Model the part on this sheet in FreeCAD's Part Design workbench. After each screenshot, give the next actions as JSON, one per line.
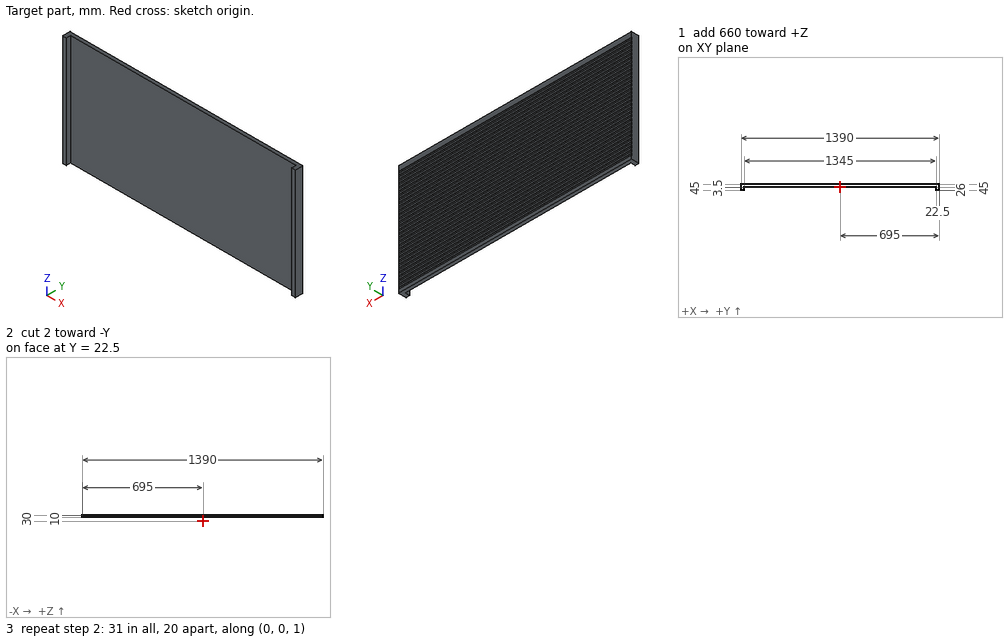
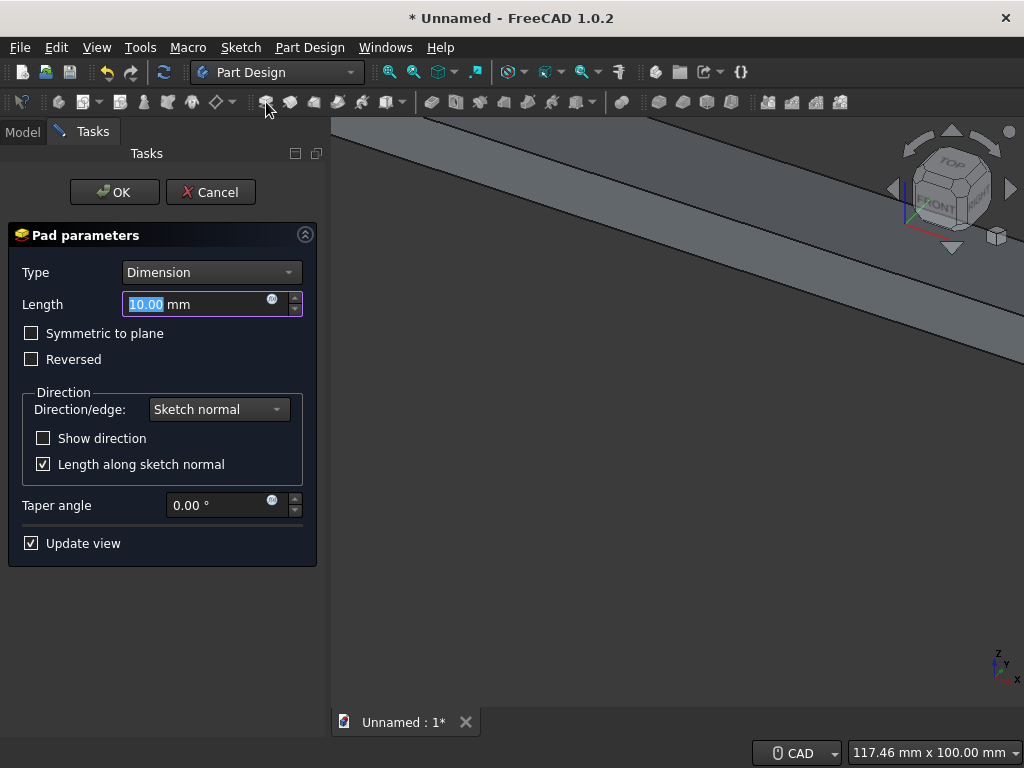
{"action": "type", "text": "660"}
{"action": "key", "text": "Tab"}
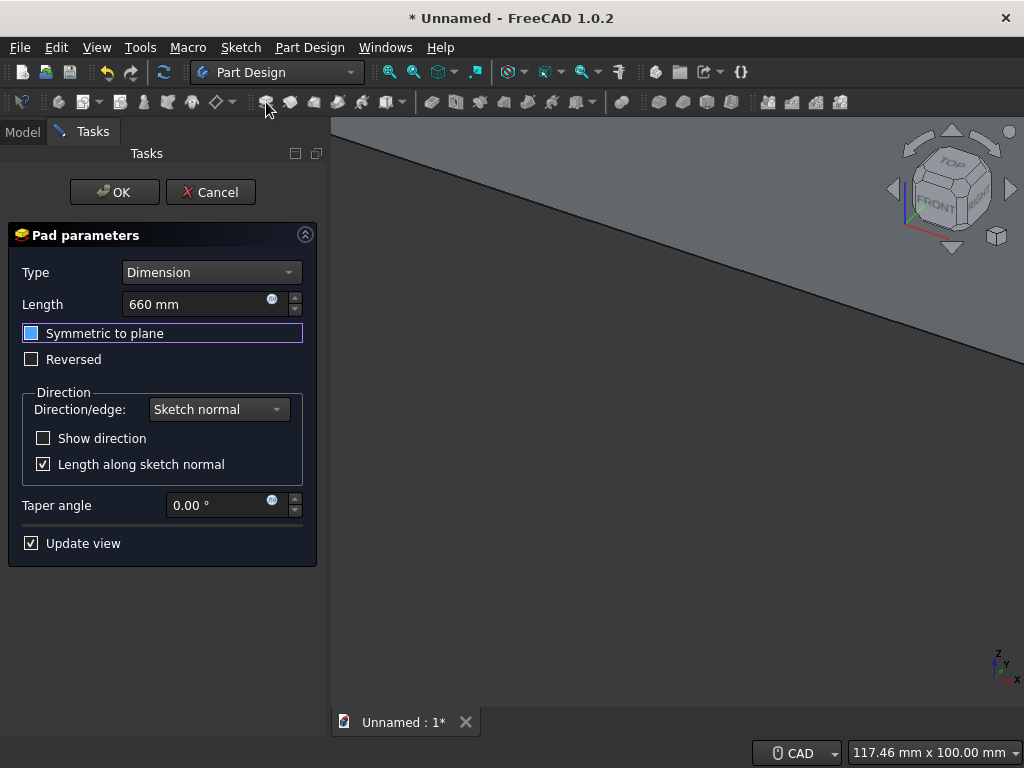
{"action": "left_click", "coordinate": [115, 192]}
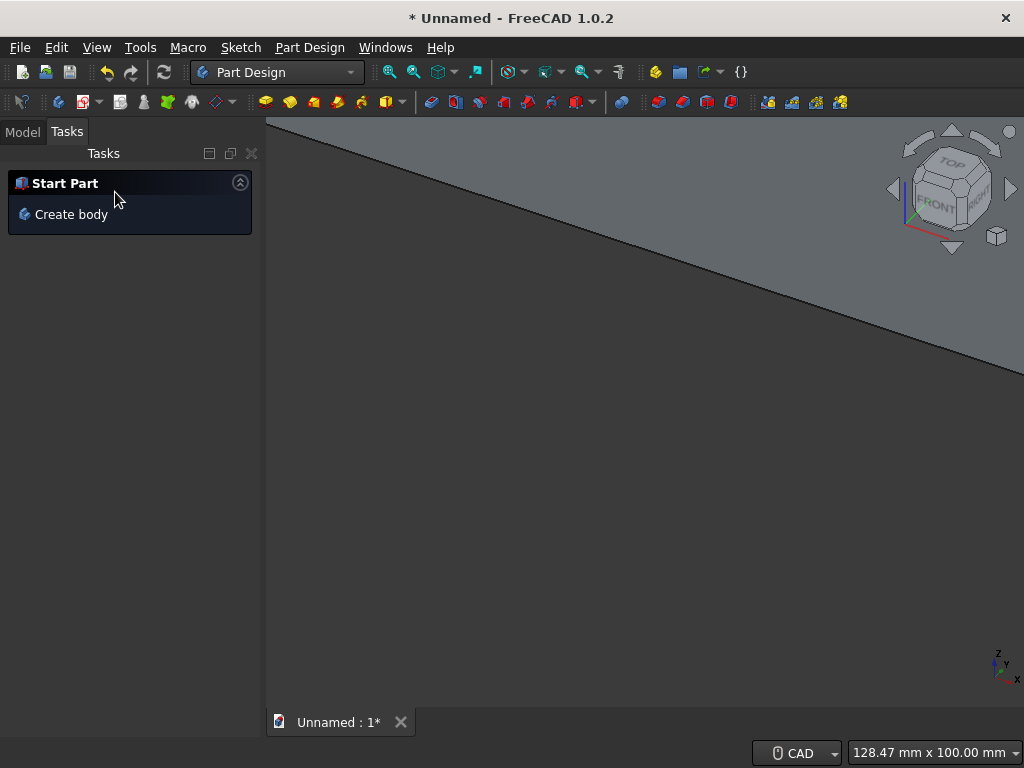
{"action": "key", "text": "v f"}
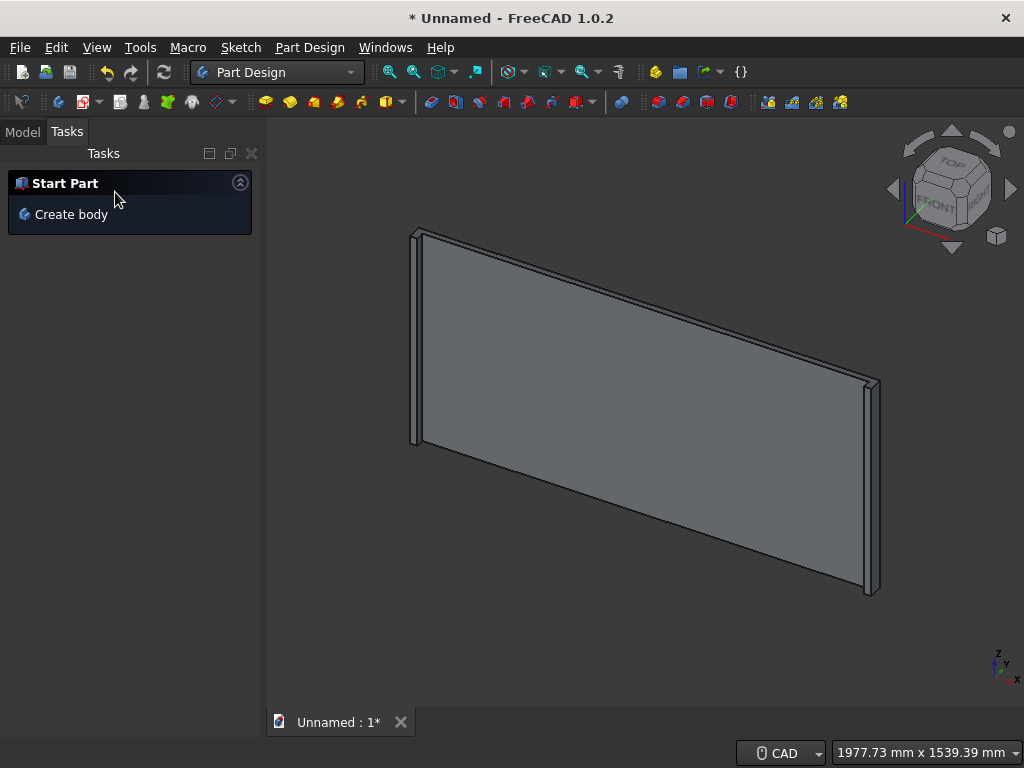
{"action": "key", "text": "4"}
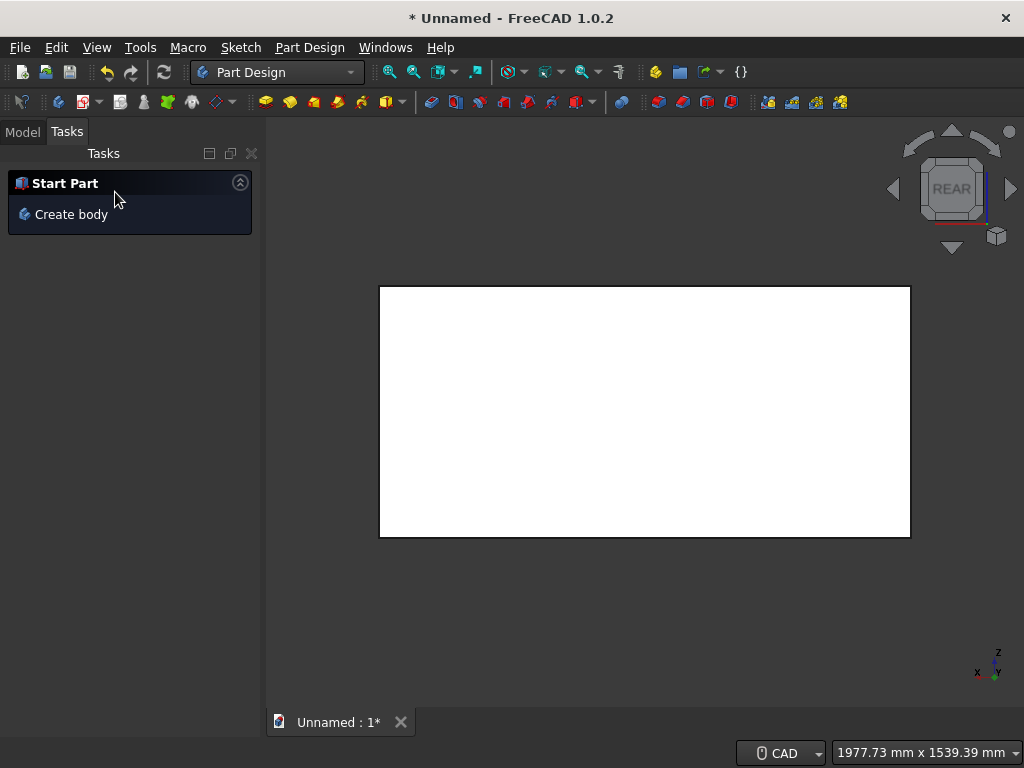
{"action": "left_click", "coordinate": [569, 411]}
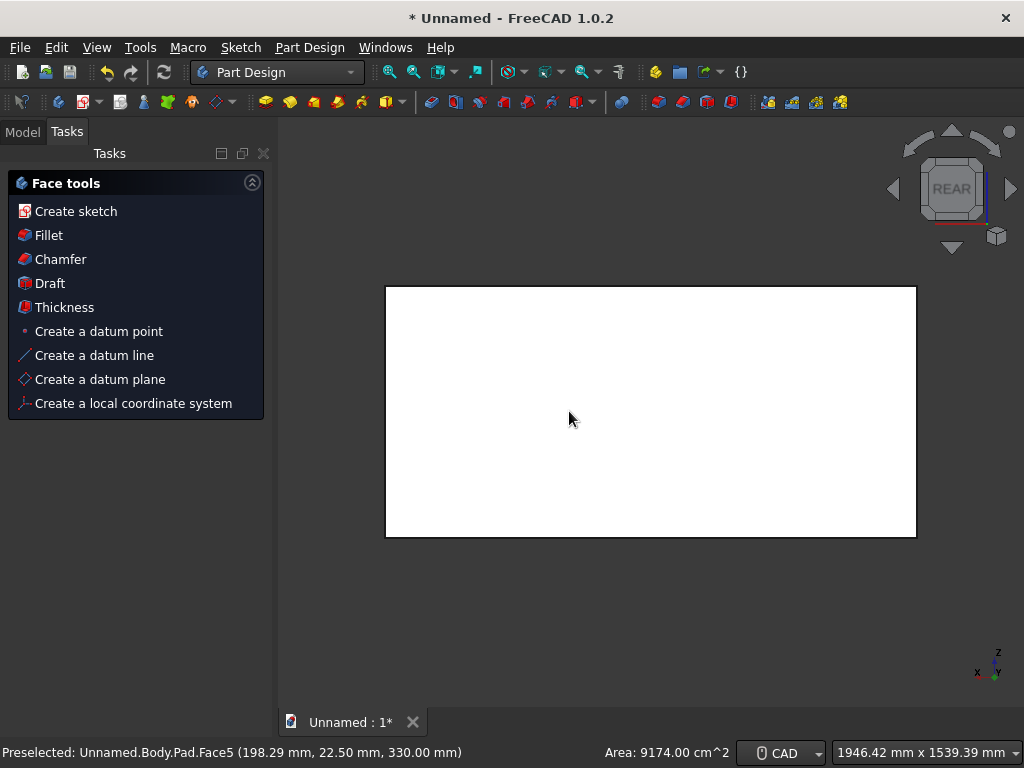
{"action": "left_click", "coordinate": [84, 102]}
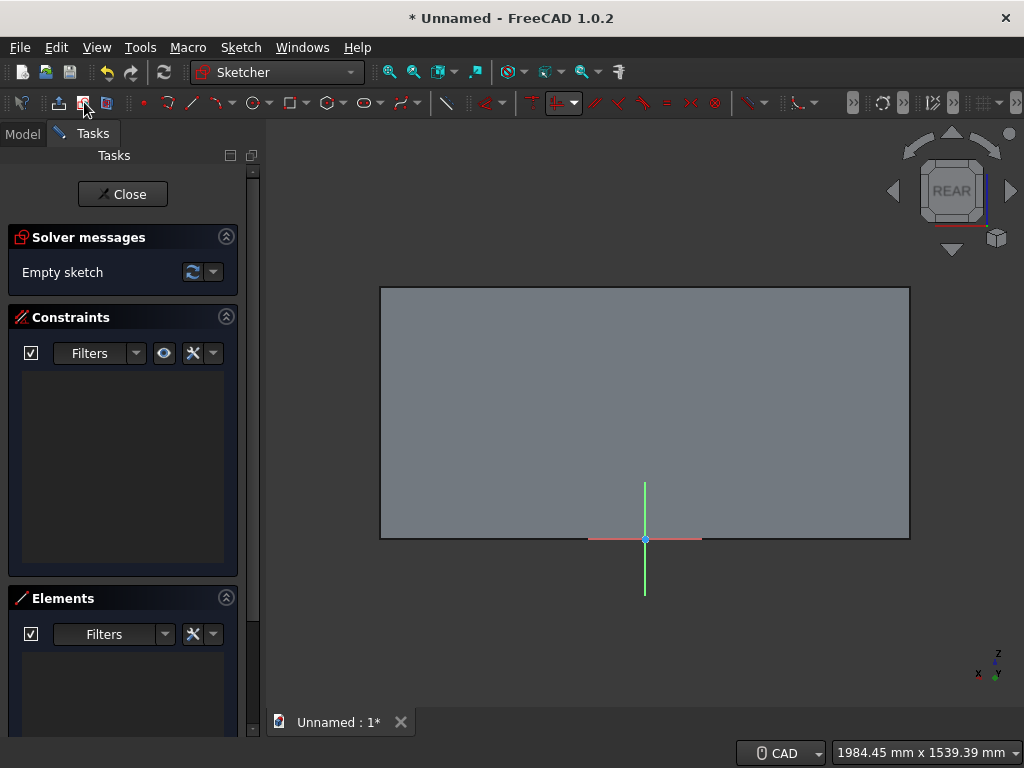
{"action": "scroll", "coordinate": [294, 147], "scroll_direction": "down", "scroll_amount": 1}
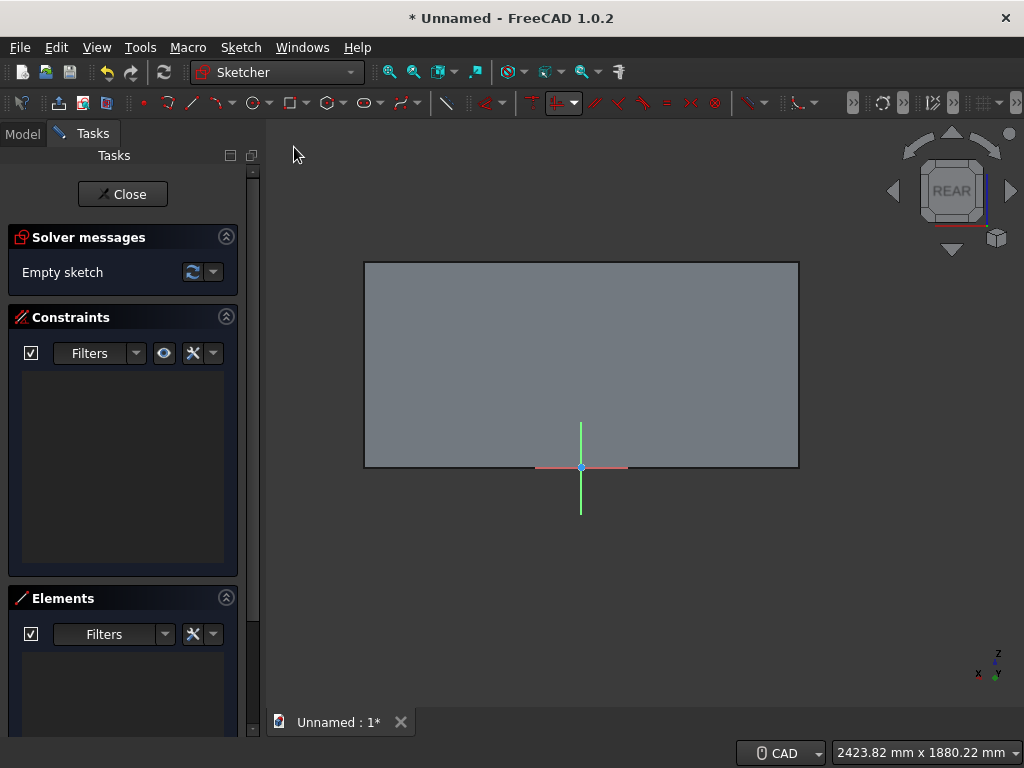
{"action": "key", "text": "g r"}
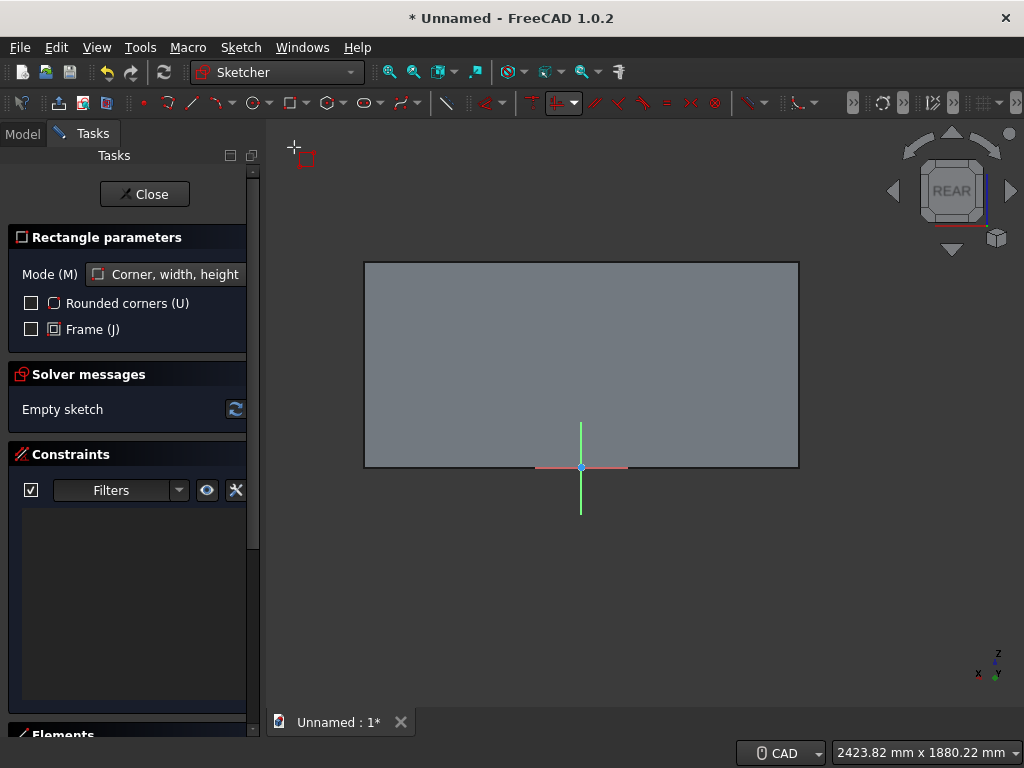
{"action": "scroll", "coordinate": [364, 459], "scroll_direction": "up", "scroll_amount": 9}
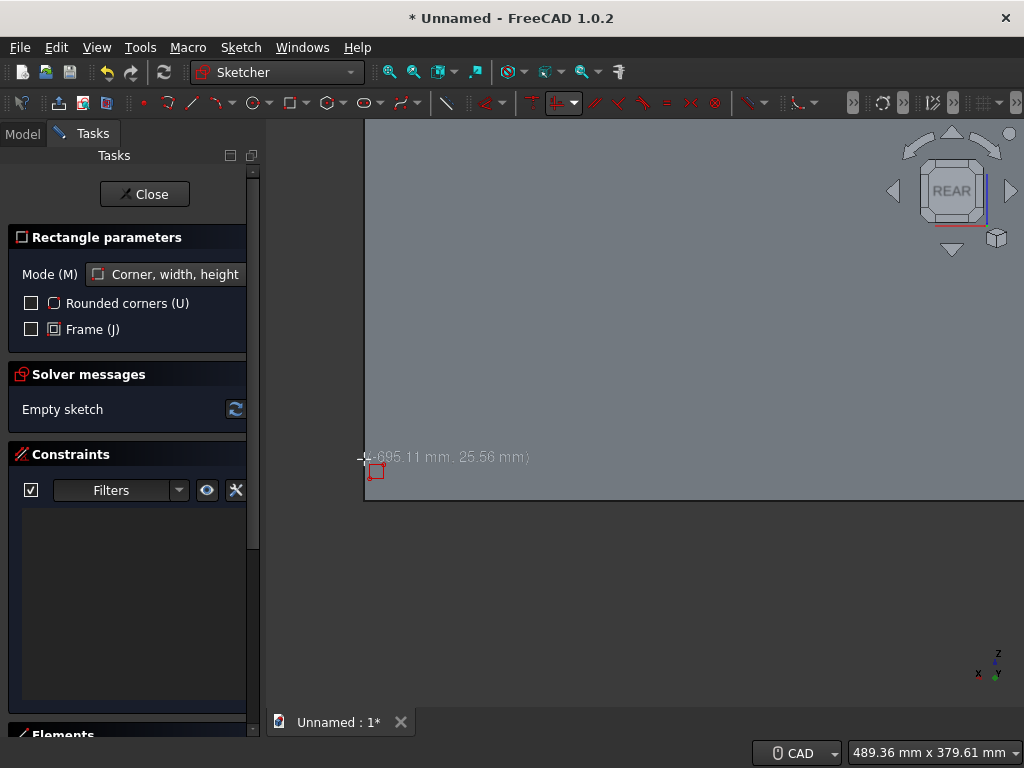
{"action": "scroll", "coordinate": [358, 399], "scroll_direction": "down", "scroll_amount": 9}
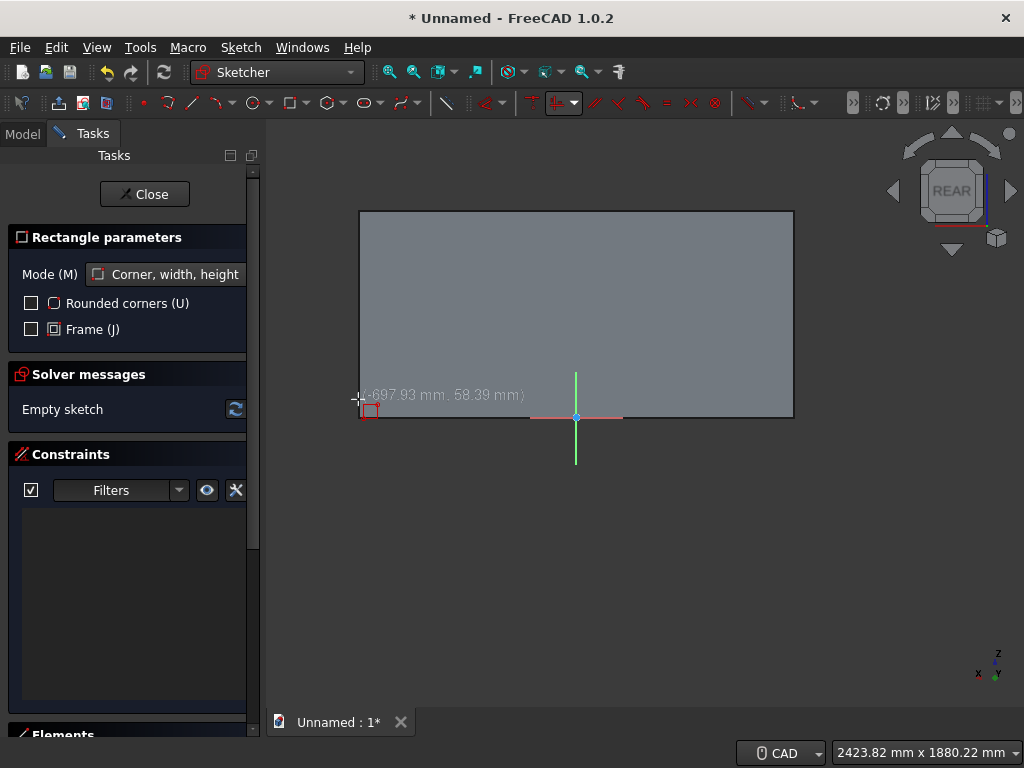
{"action": "scroll", "coordinate": [359, 408], "scroll_direction": "up", "scroll_amount": 3}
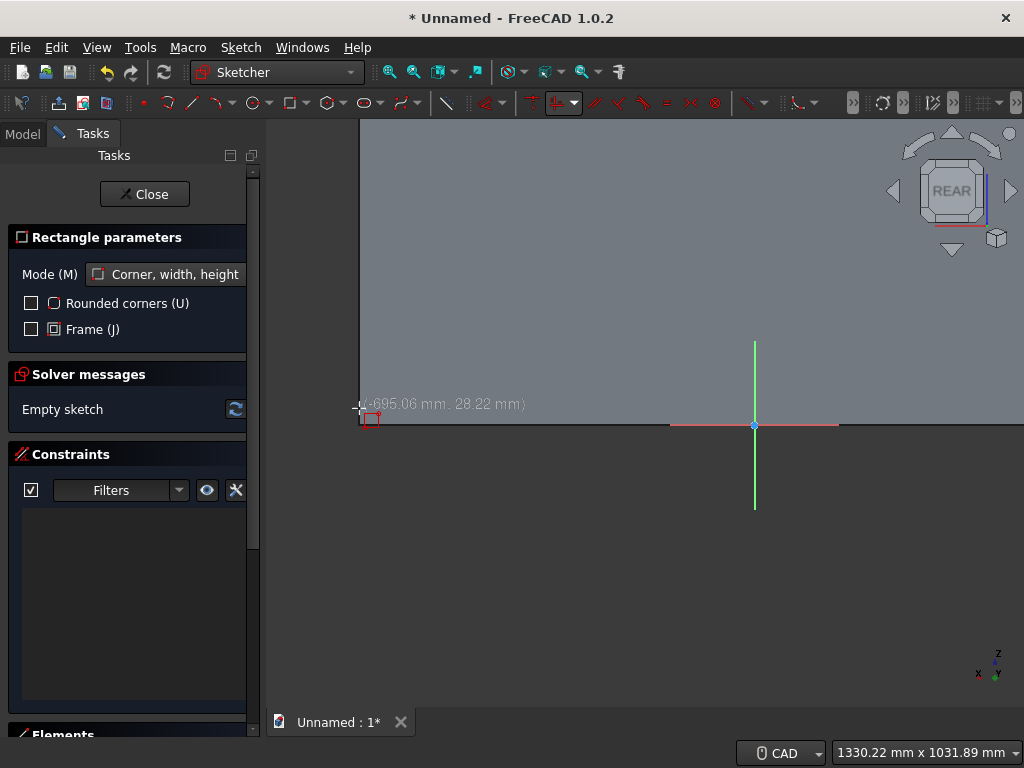
{"action": "left_click", "coordinate": [359, 408]}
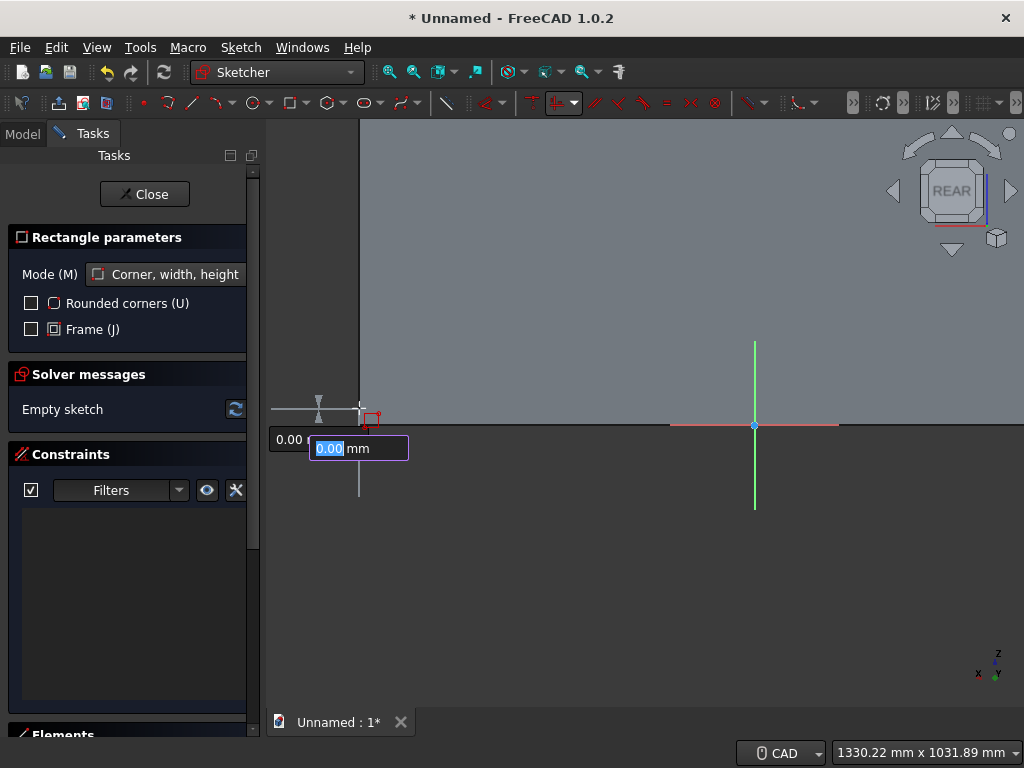
{"action": "scroll", "coordinate": [359, 408], "scroll_direction": "down", "scroll_amount": 3}